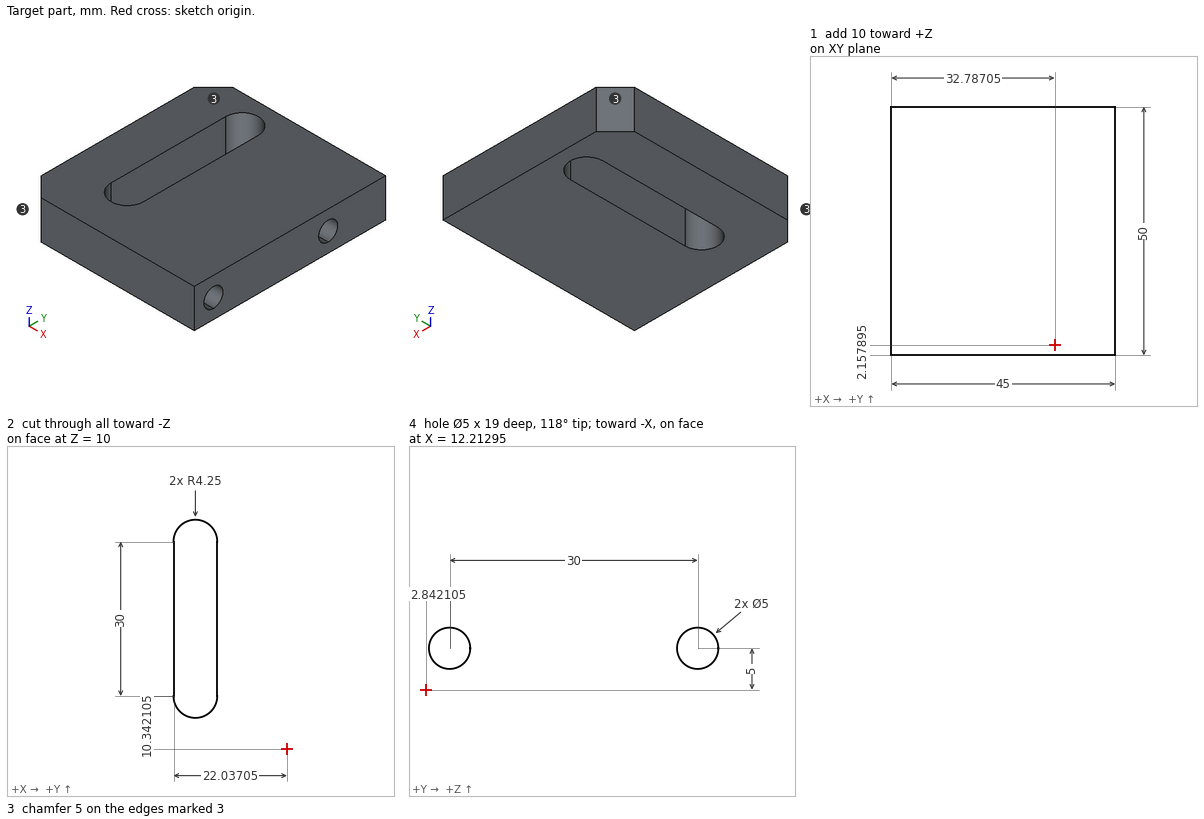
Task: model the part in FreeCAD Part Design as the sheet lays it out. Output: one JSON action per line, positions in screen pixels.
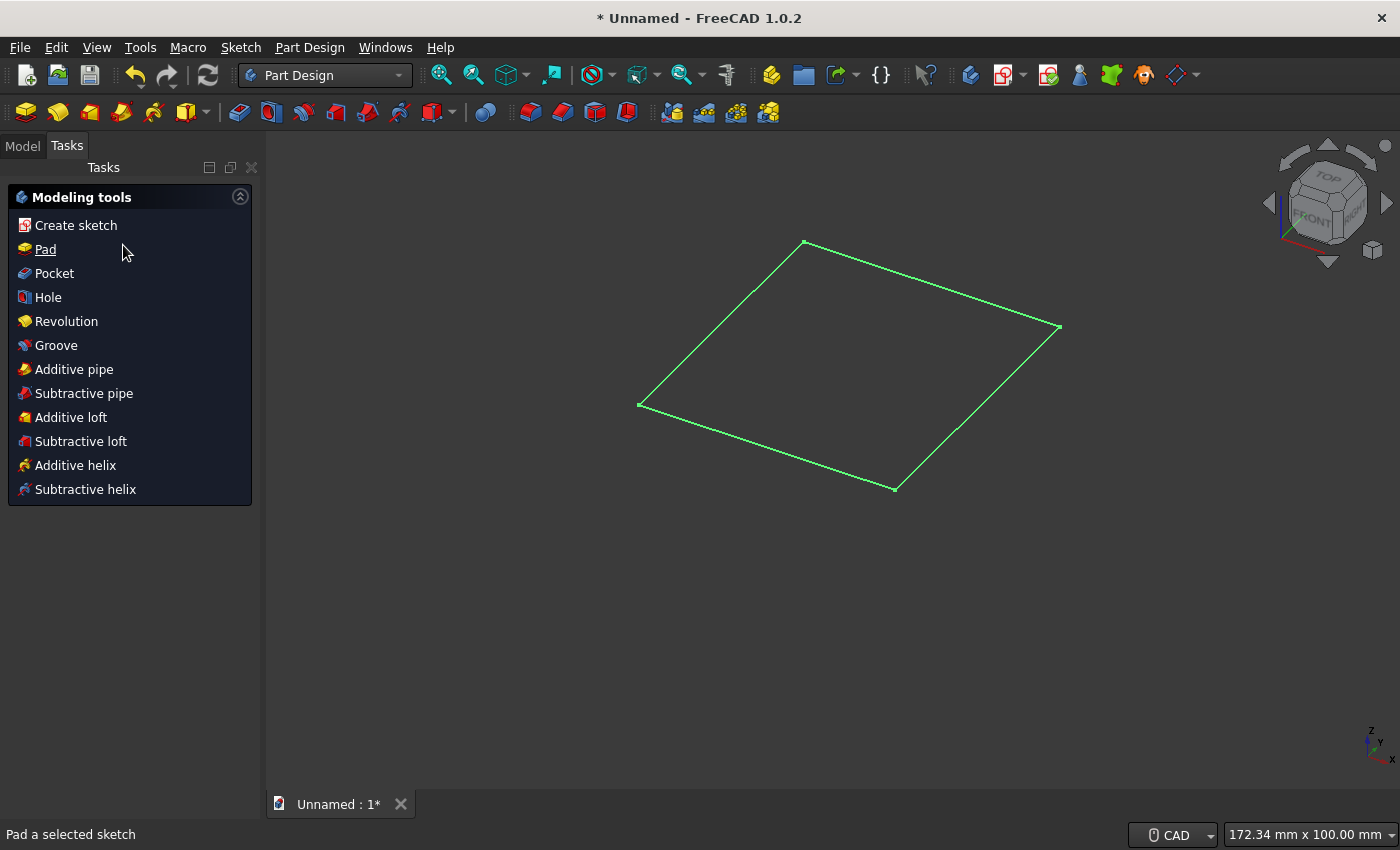
{"action": "left_click", "coordinate": [26, 112]}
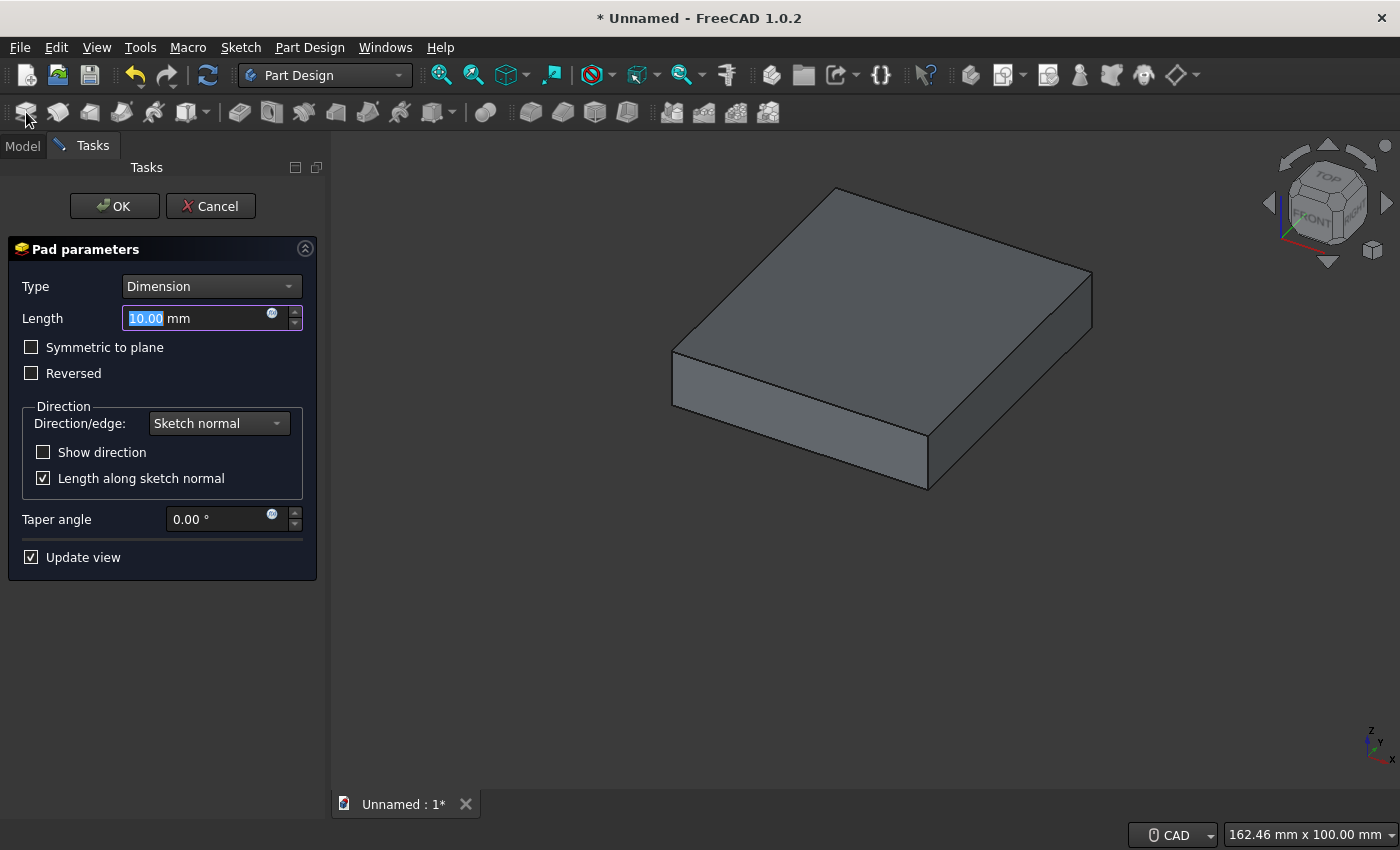
{"action": "type", "text": "10"}
{"action": "key", "text": "Tab"}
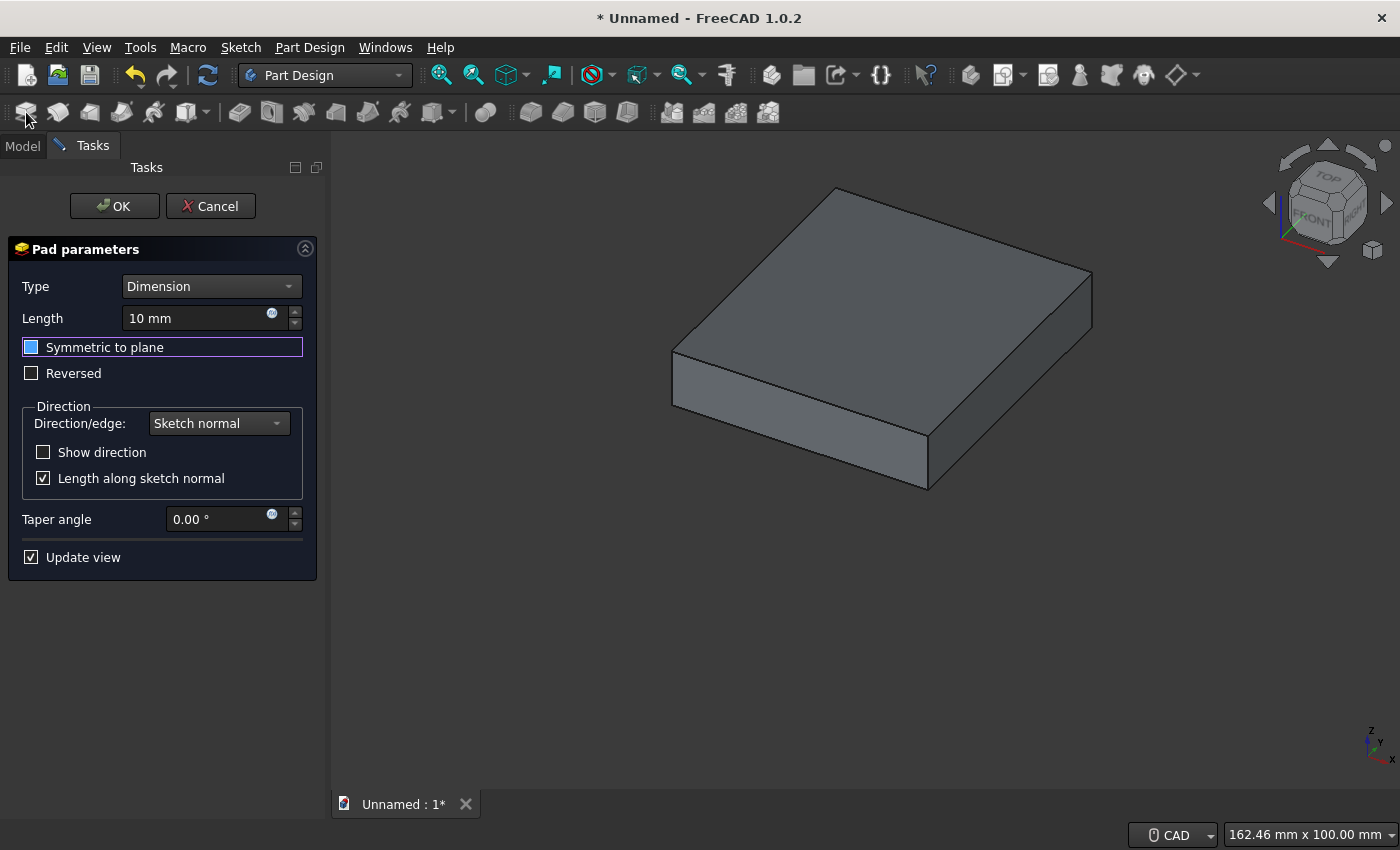
{"action": "left_click", "coordinate": [115, 206]}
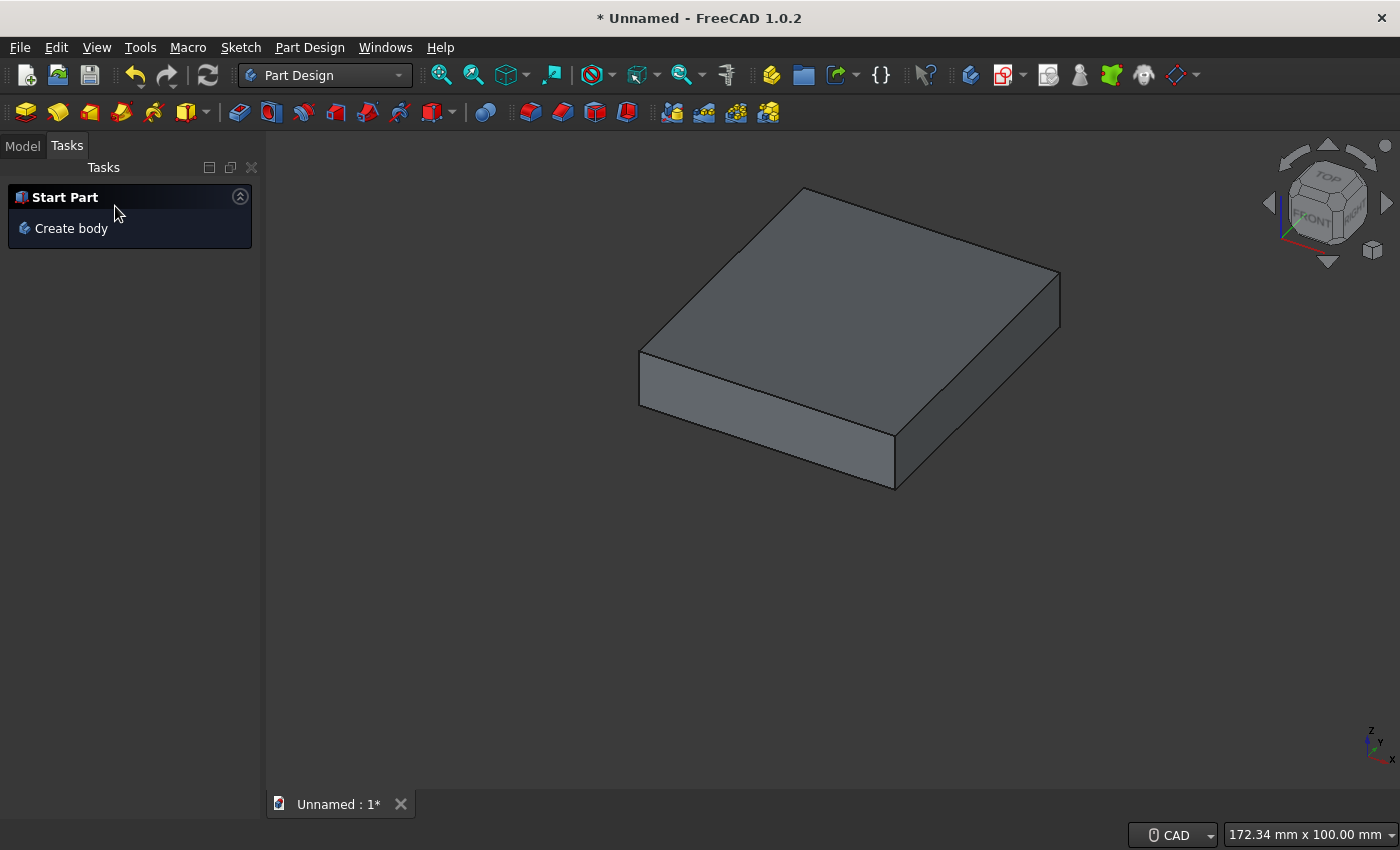
{"action": "left_click", "coordinate": [850, 311]}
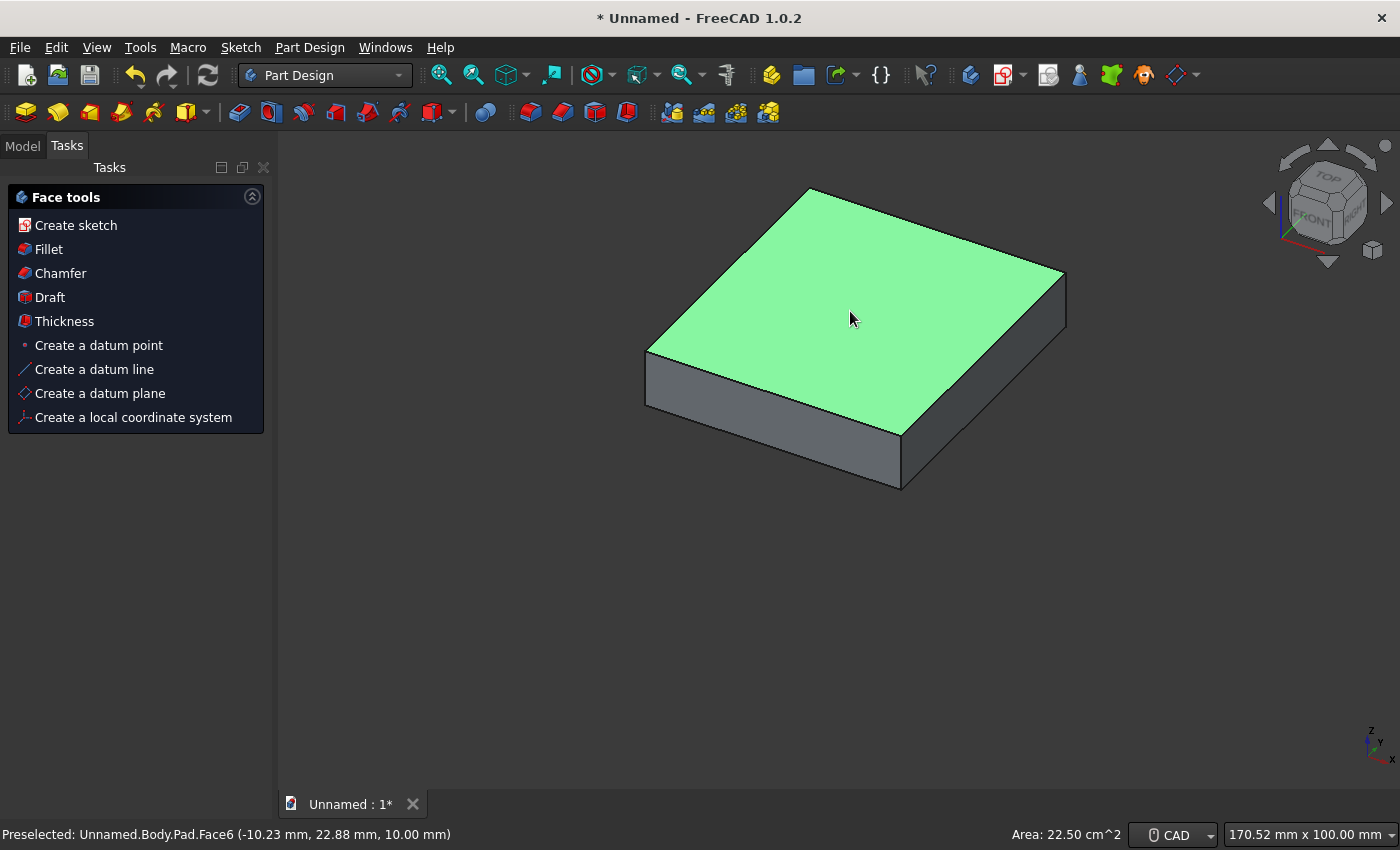
{"action": "left_click", "coordinate": [1004, 76]}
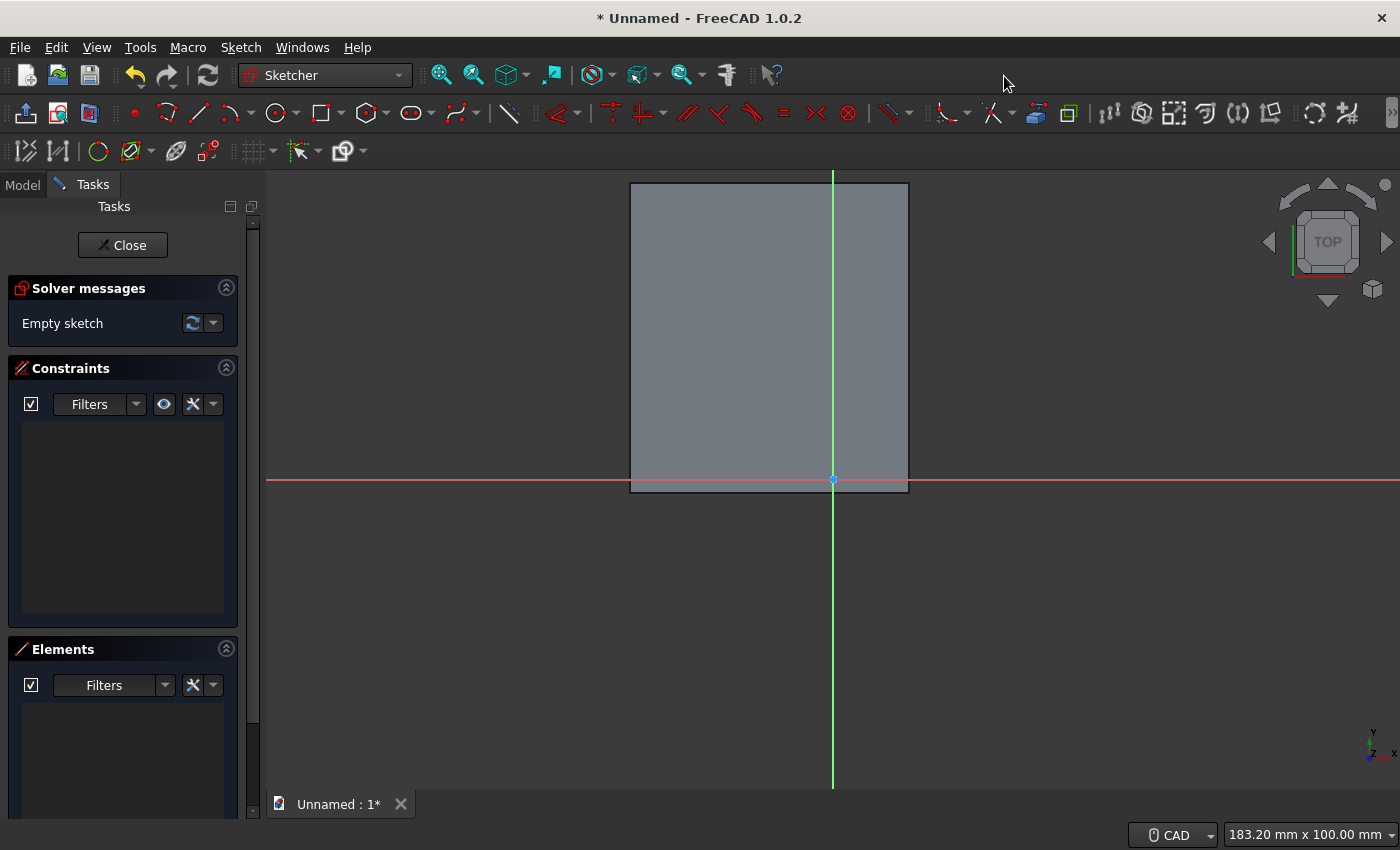
{"action": "scroll", "coordinate": [763, 761], "scroll_direction": "down", "scroll_amount": 1}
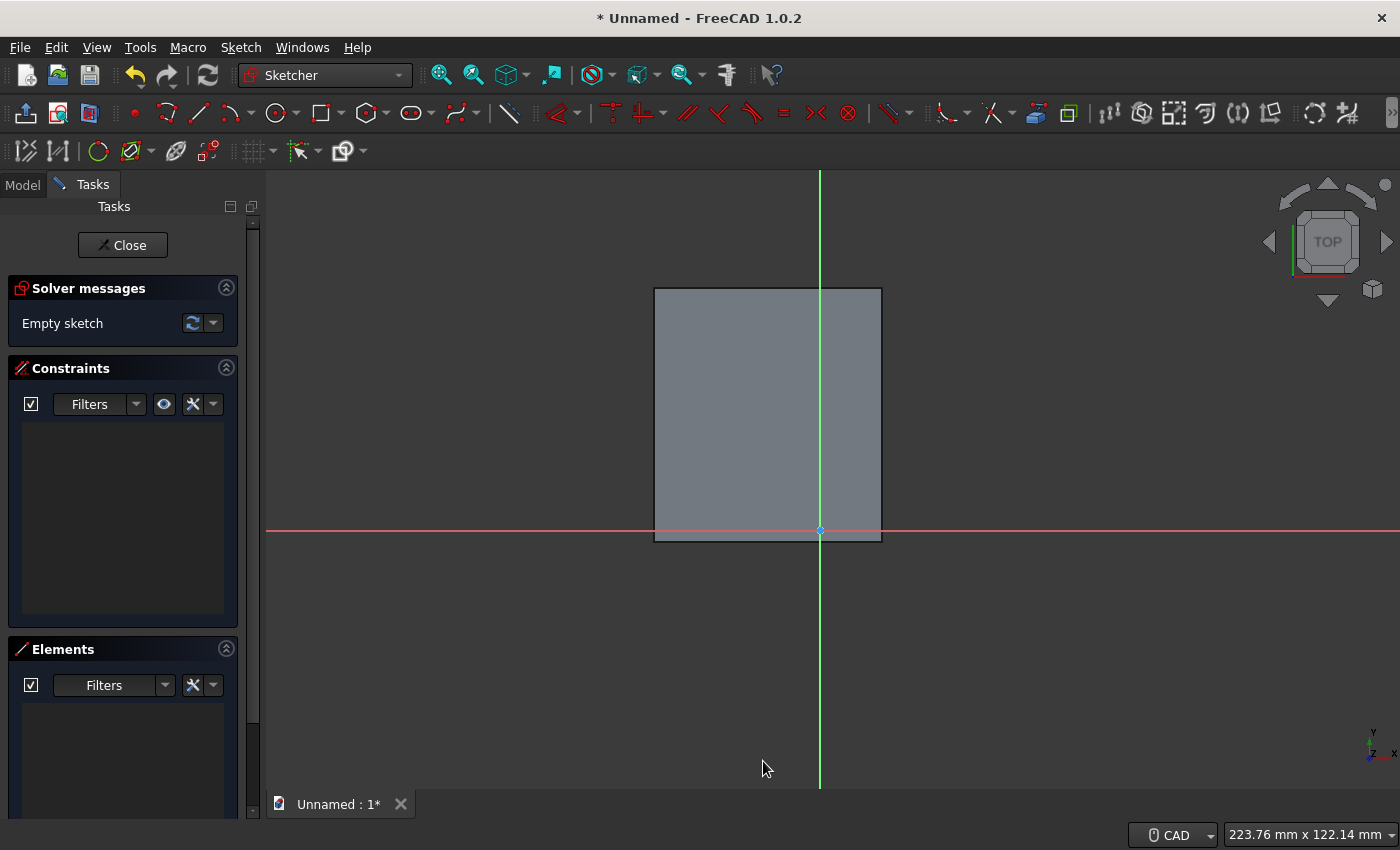
{"action": "scroll", "coordinate": [765, 343], "scroll_direction": "up", "scroll_amount": 3}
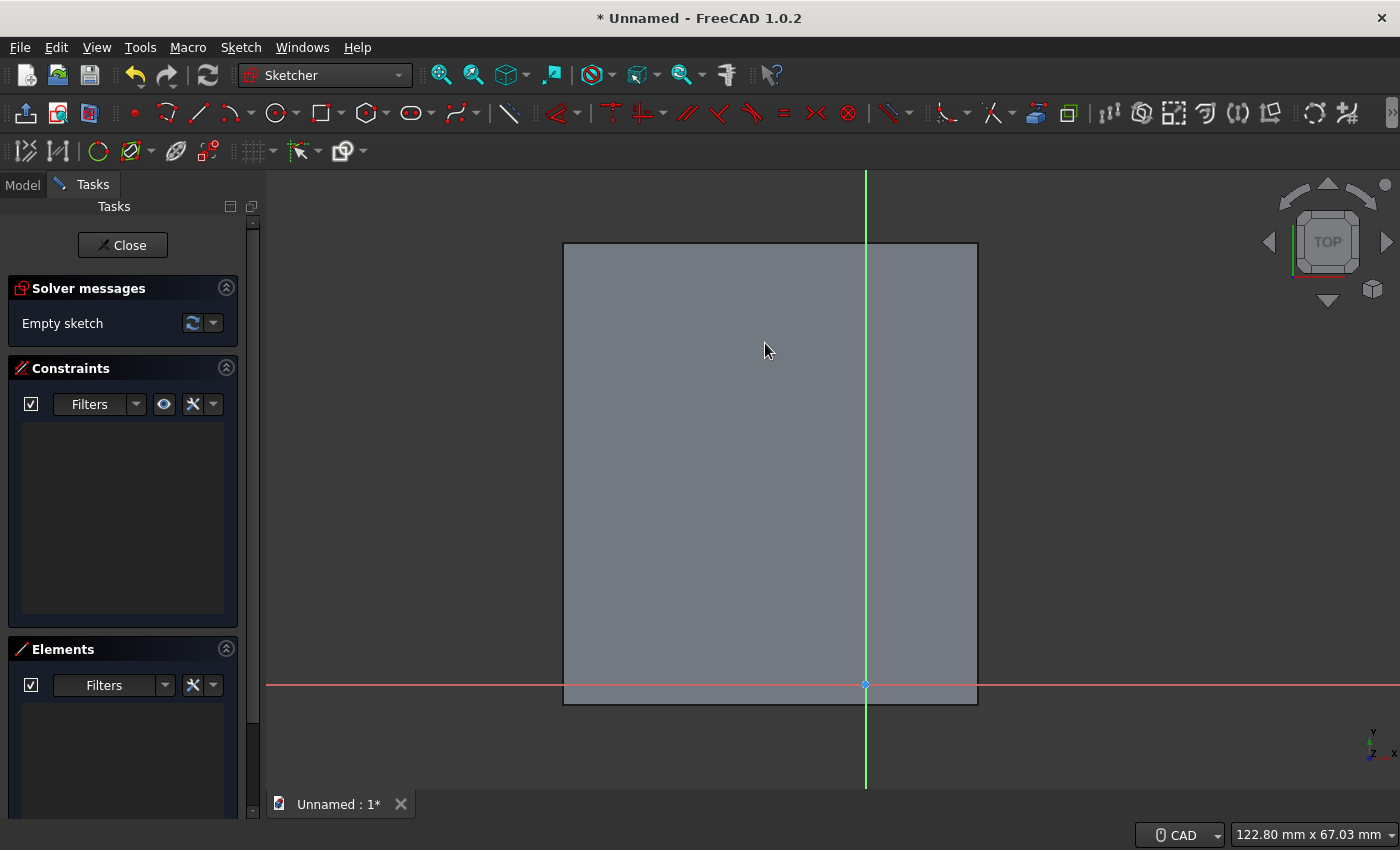
{"action": "left_click", "coordinate": [412, 114]}